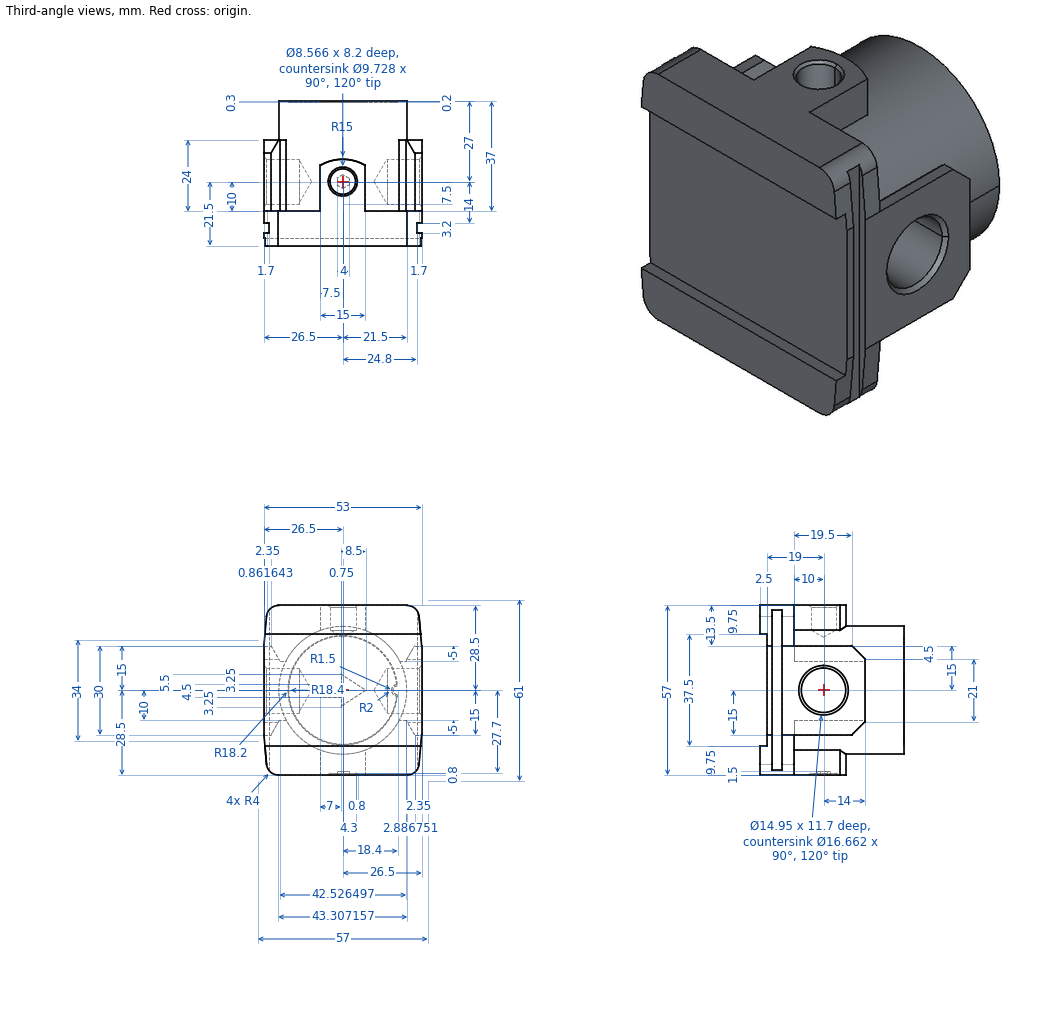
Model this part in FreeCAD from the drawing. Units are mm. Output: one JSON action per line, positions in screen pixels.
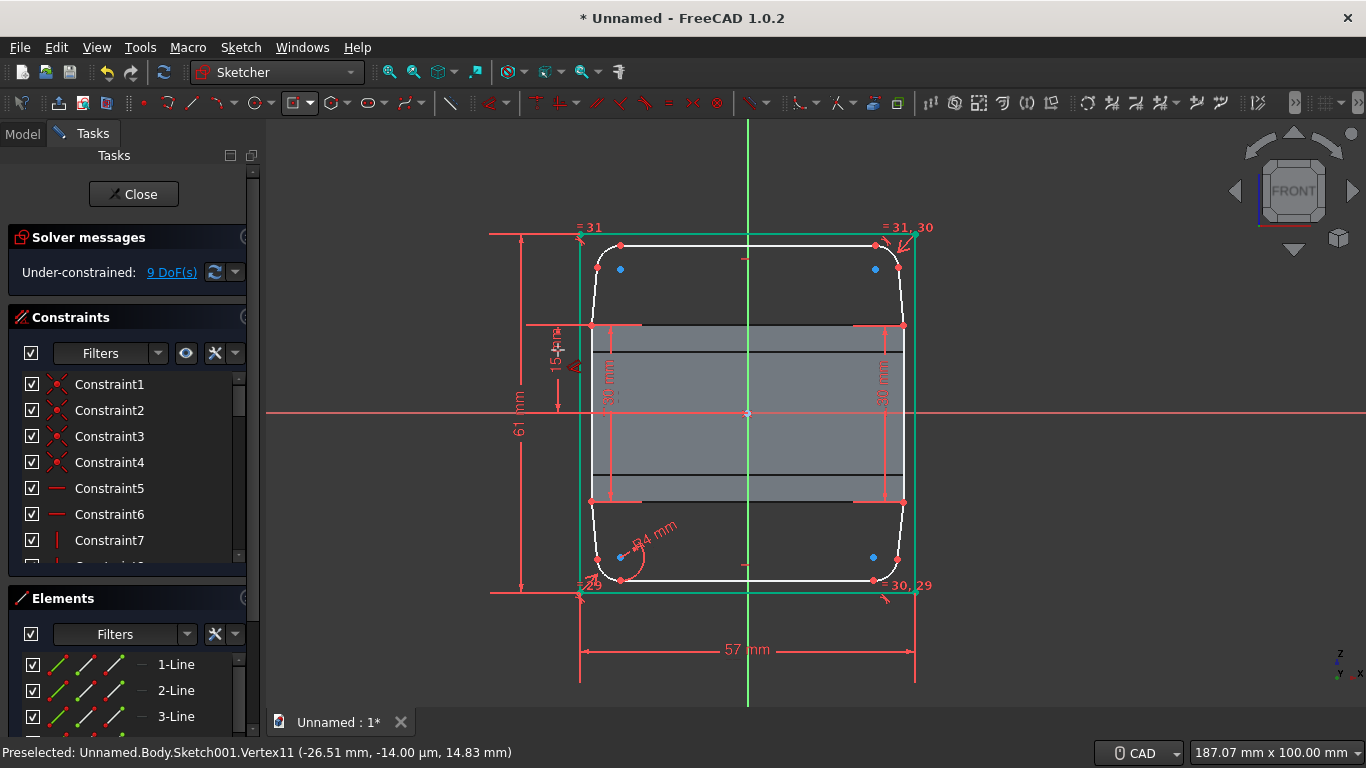
{"action": "left_click", "coordinate": [904, 502]}
{"action": "left_click", "coordinate": [938, 458]}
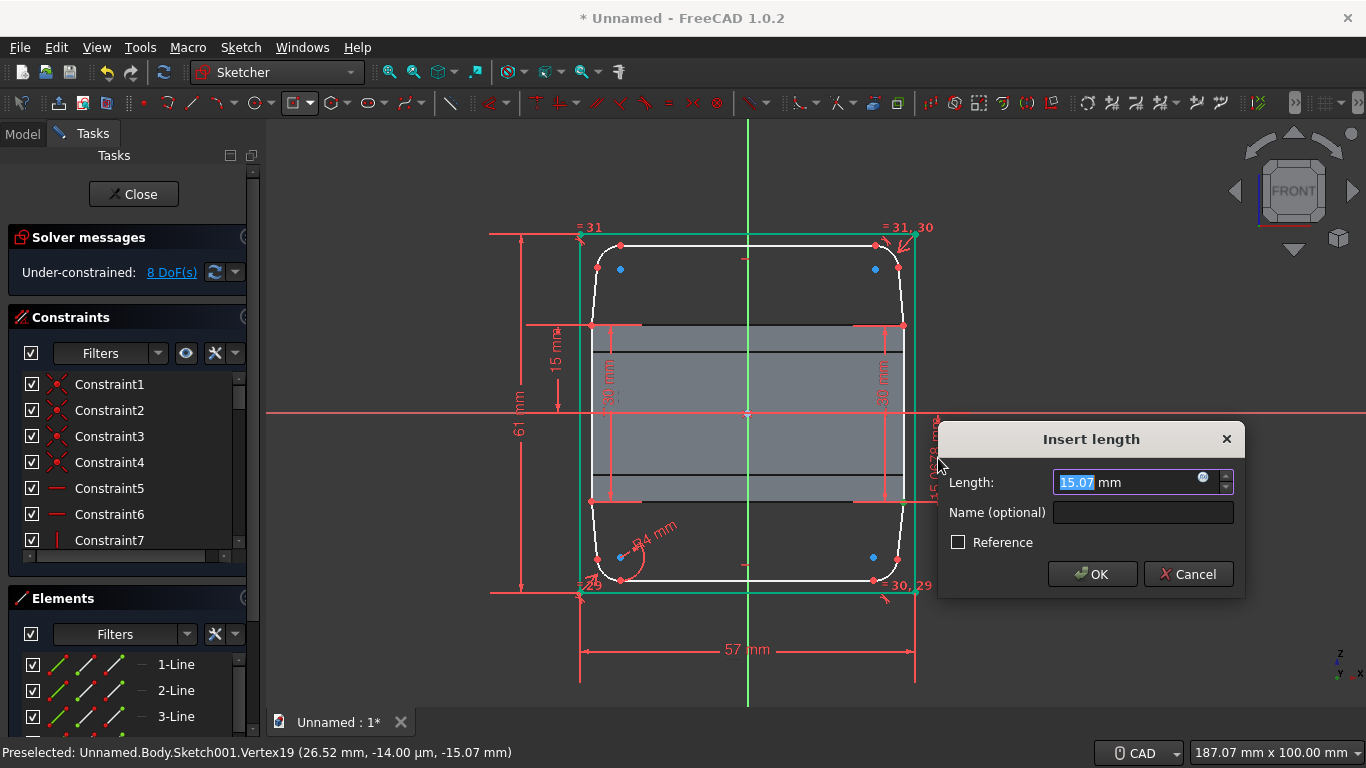
{"action": "type", "text": "15"}
{"action": "key", "text": "Return"}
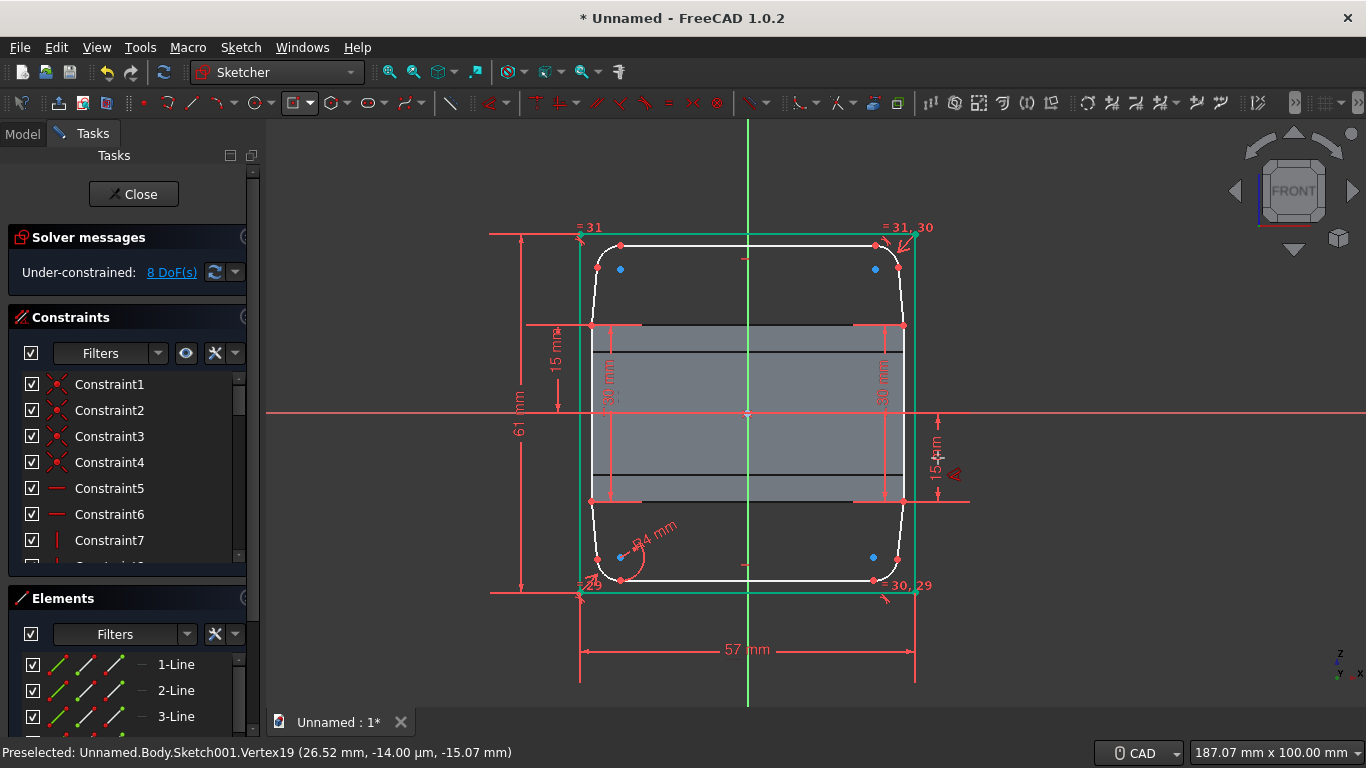
{"action": "left_click", "coordinate": [592, 325]}
{"action": "left_click", "coordinate": [670, 291]}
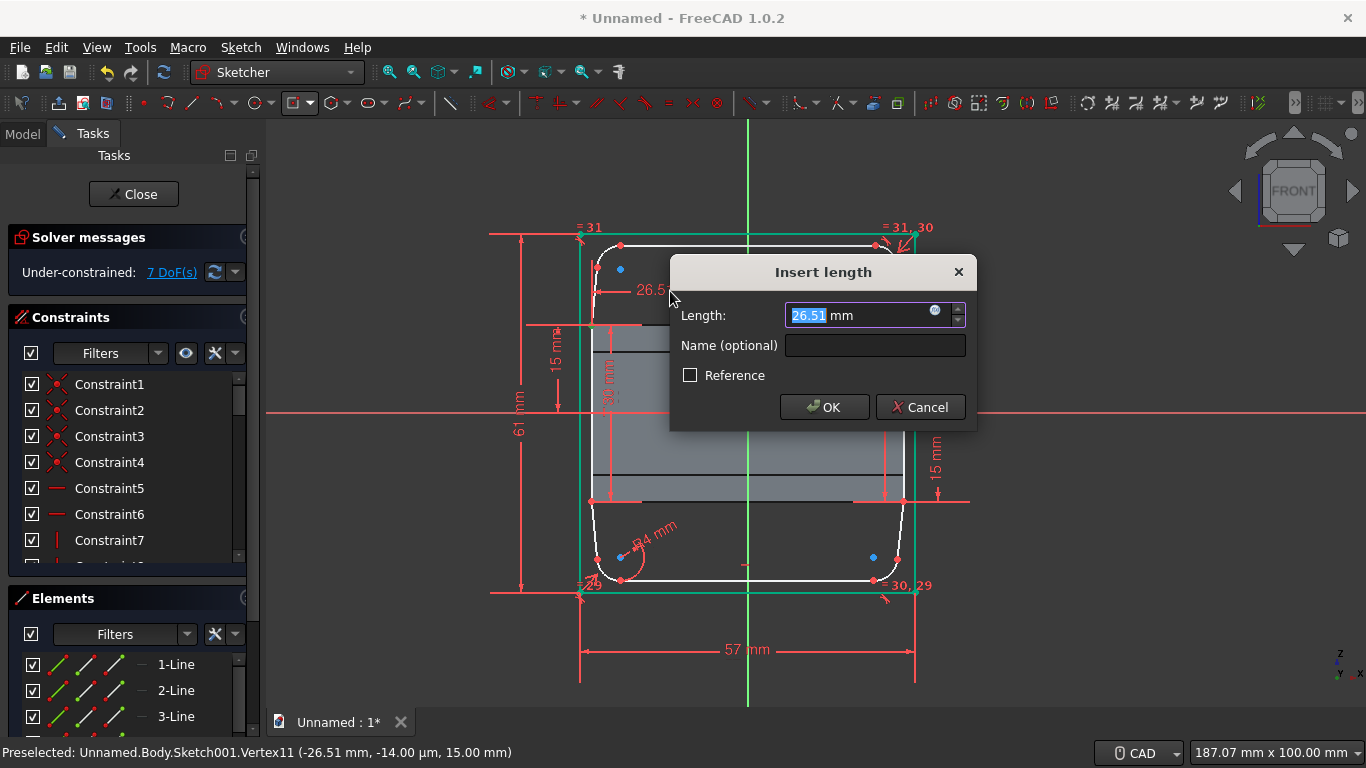
{"action": "type", "text": "26.5"}
{"action": "key", "text": "Return"}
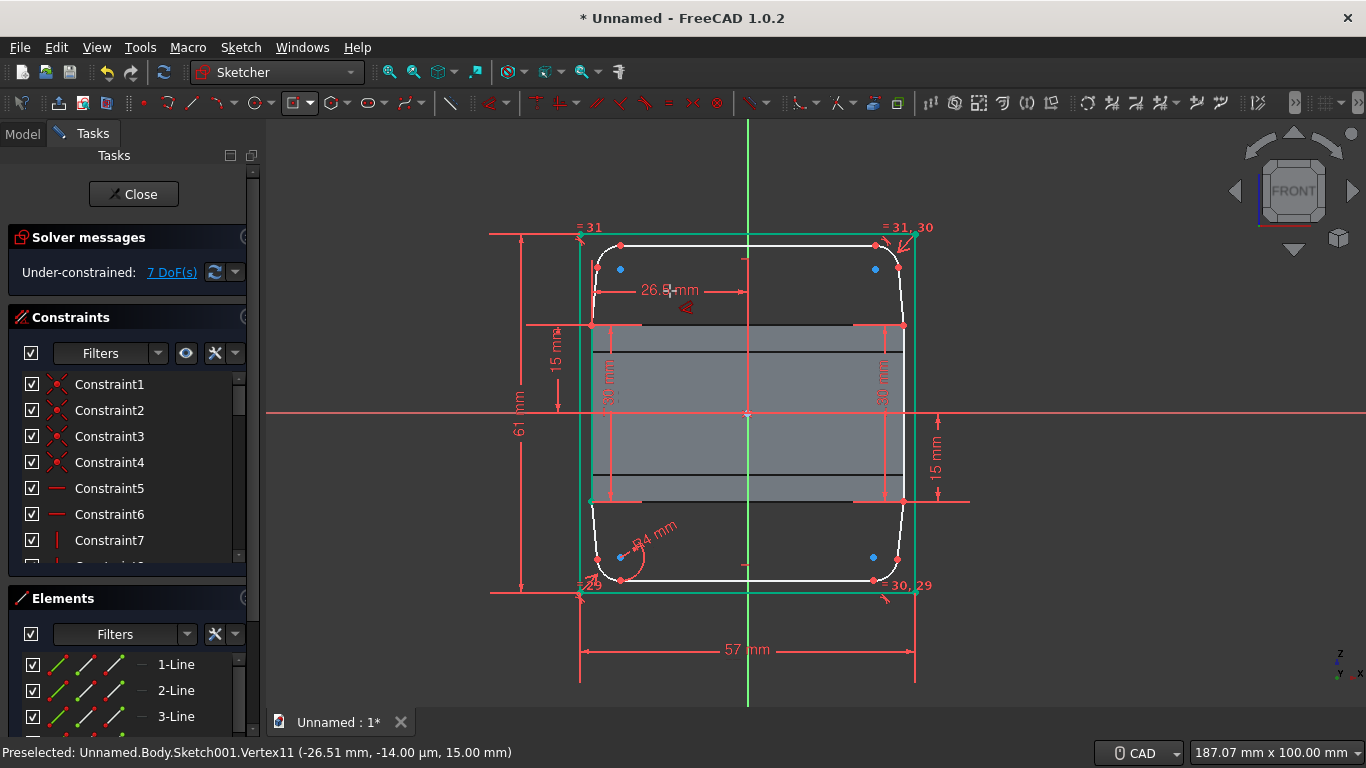
{"action": "left_click", "coordinate": [621, 581]}
{"action": "left_click", "coordinate": [782, 497]}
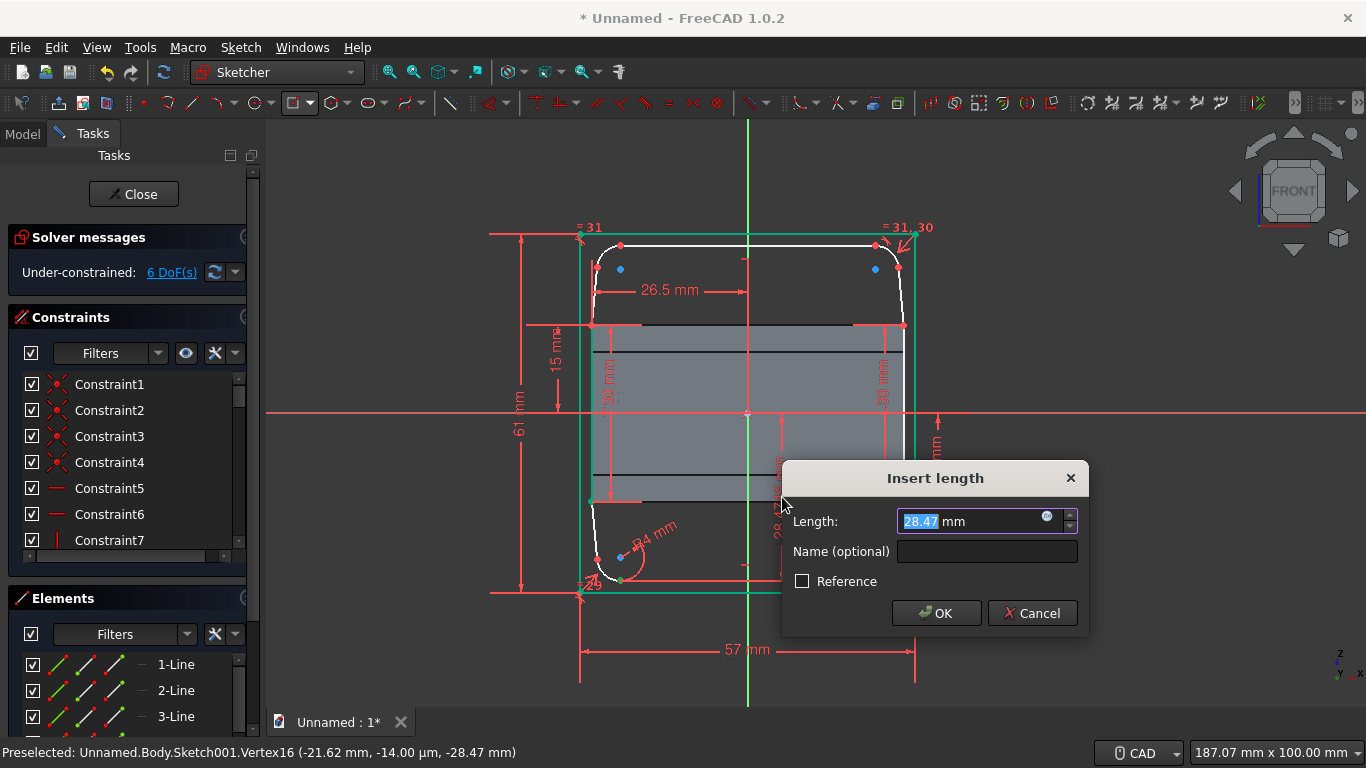
{"action": "type", "text": "28.5"}
{"action": "key", "text": "Return"}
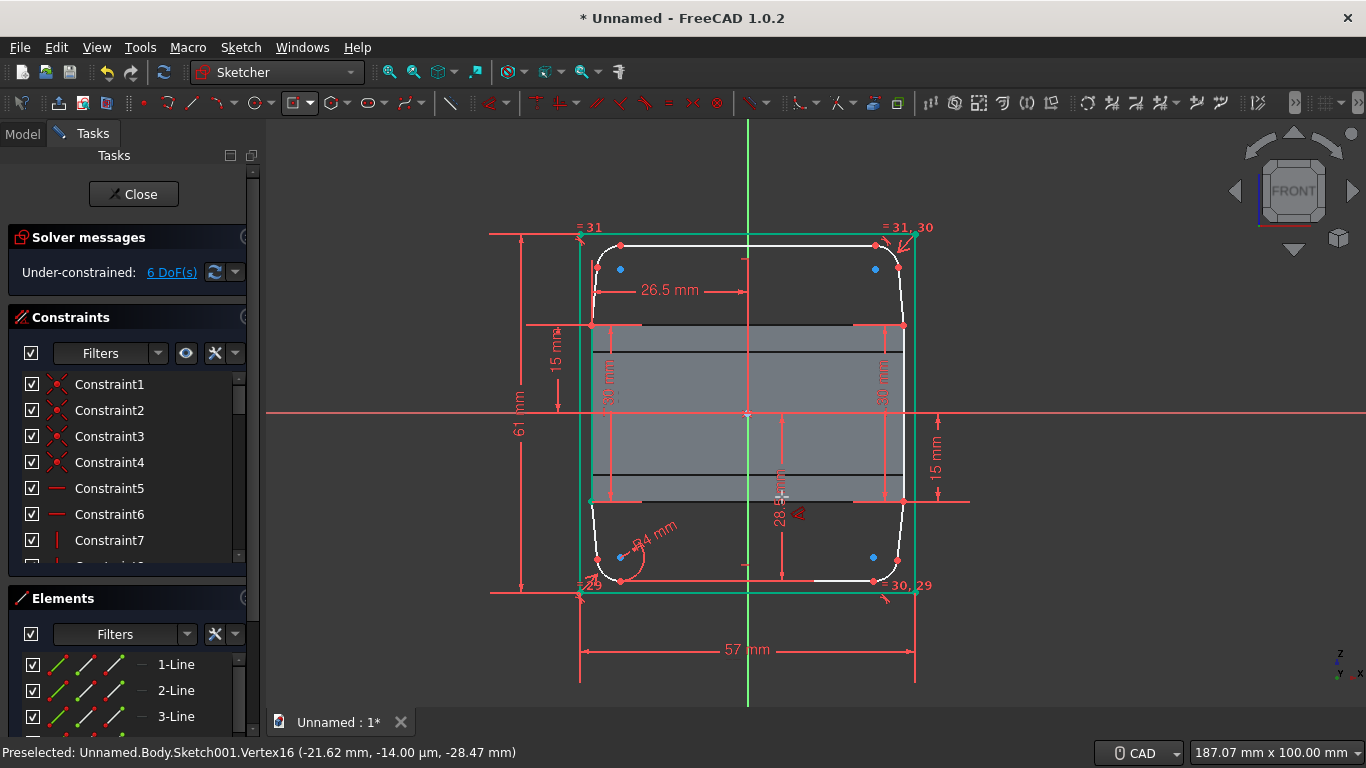
{"action": "left_click", "coordinate": [904, 502]}
{"action": "left_click", "coordinate": [826, 536]}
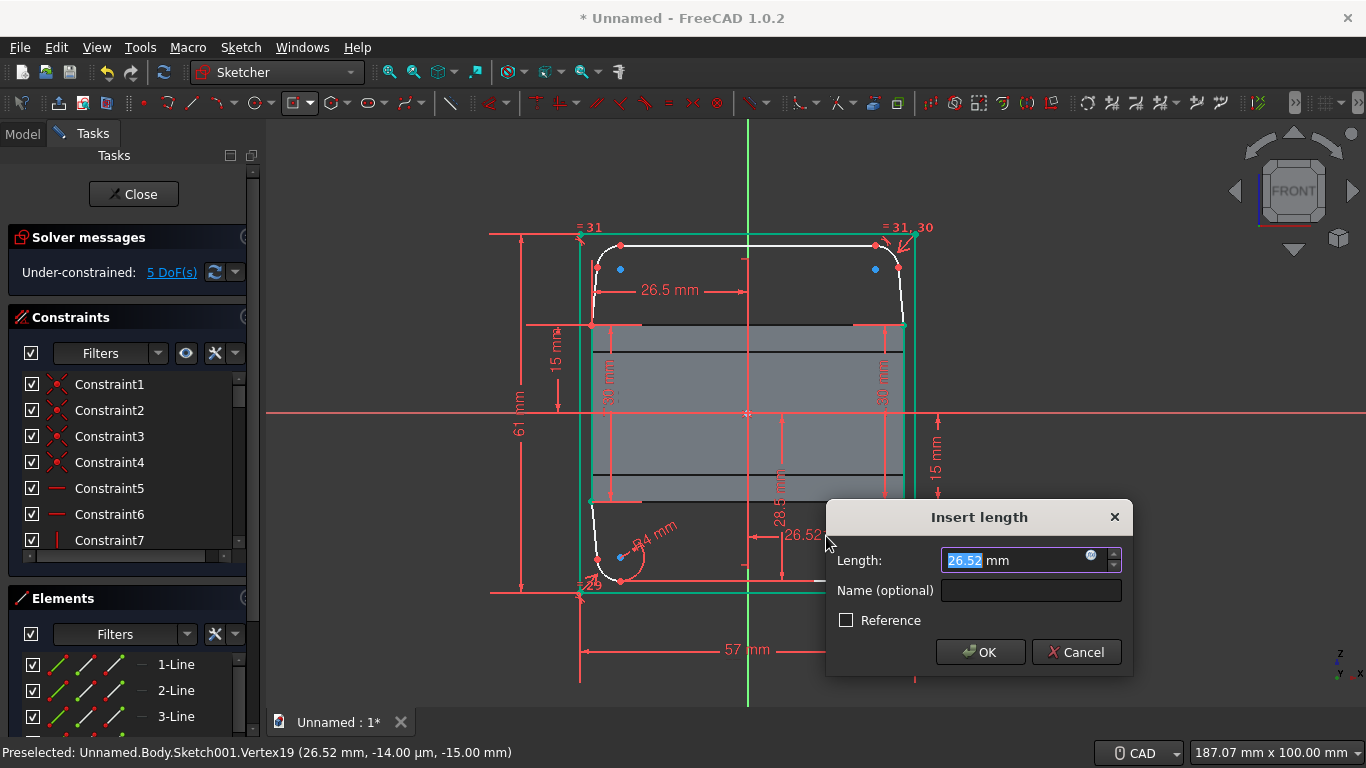
{"action": "type", "text": "26.5"}
{"action": "key", "text": "Return"}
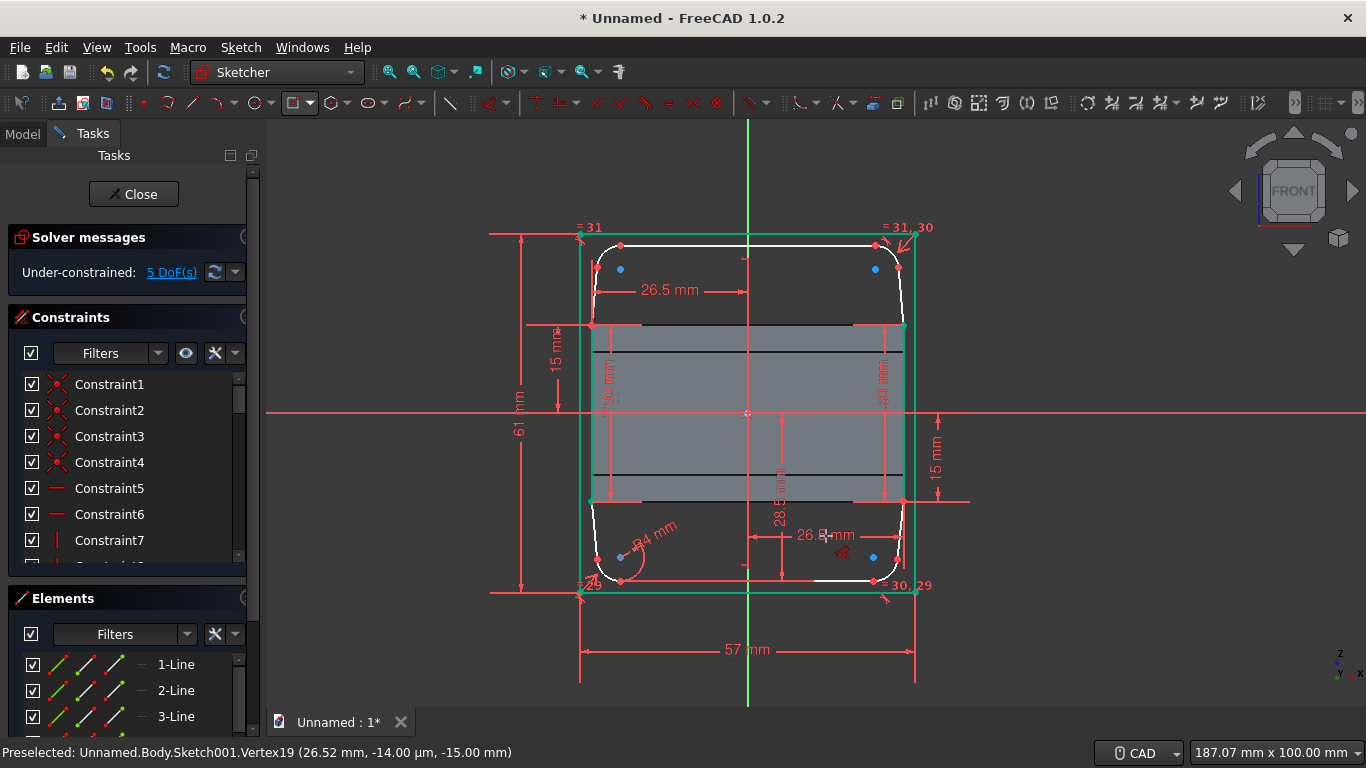
{"action": "left_click", "coordinate": [875, 246]}
{"action": "left_click", "coordinate": [714, 330]}